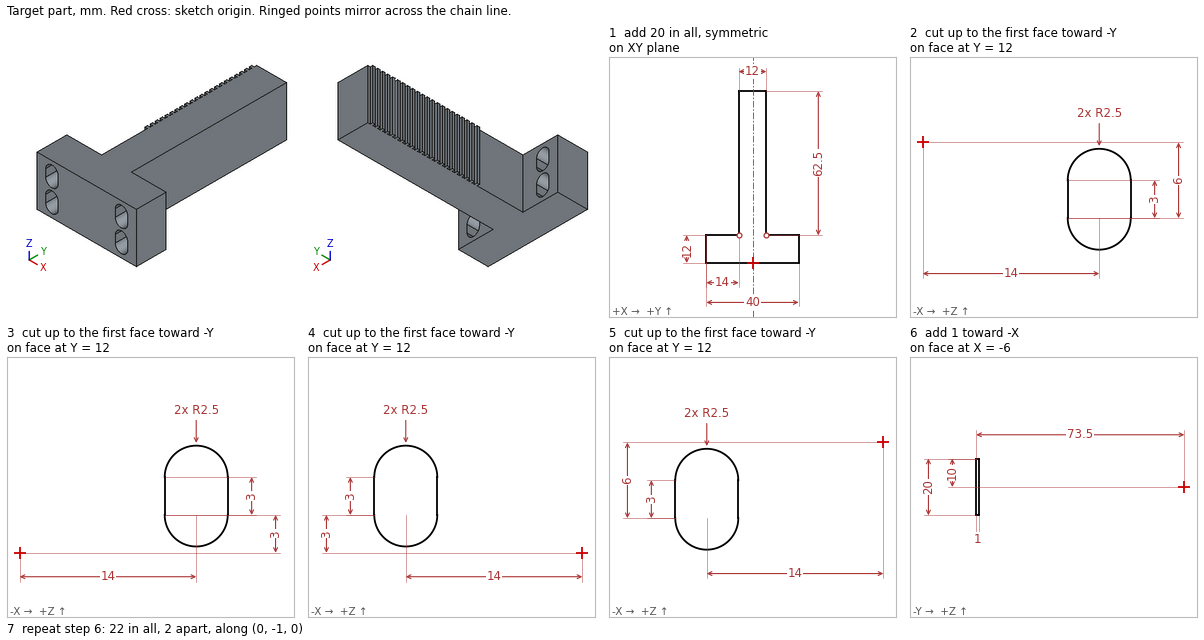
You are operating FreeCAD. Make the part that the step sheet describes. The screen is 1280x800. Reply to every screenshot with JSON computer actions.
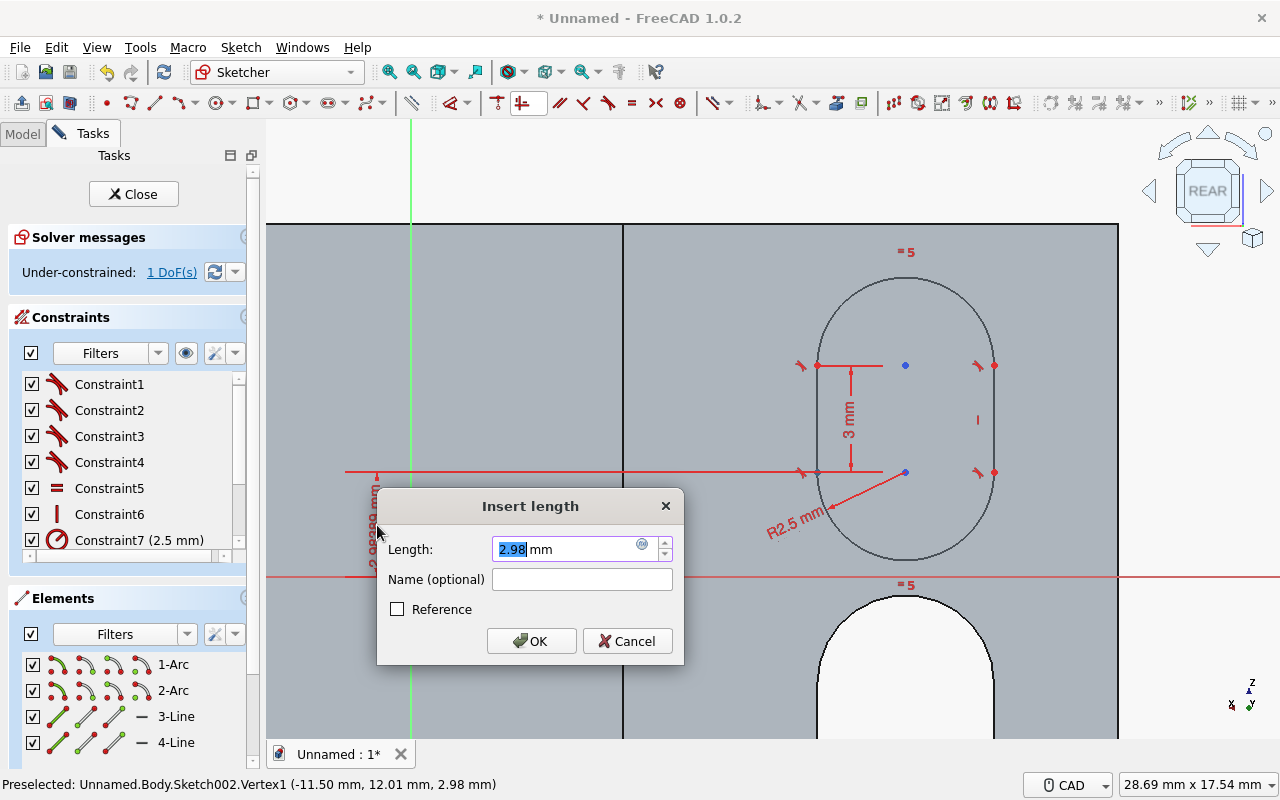
{"action": "type", "text": "3"}
{"action": "key", "text": "Return"}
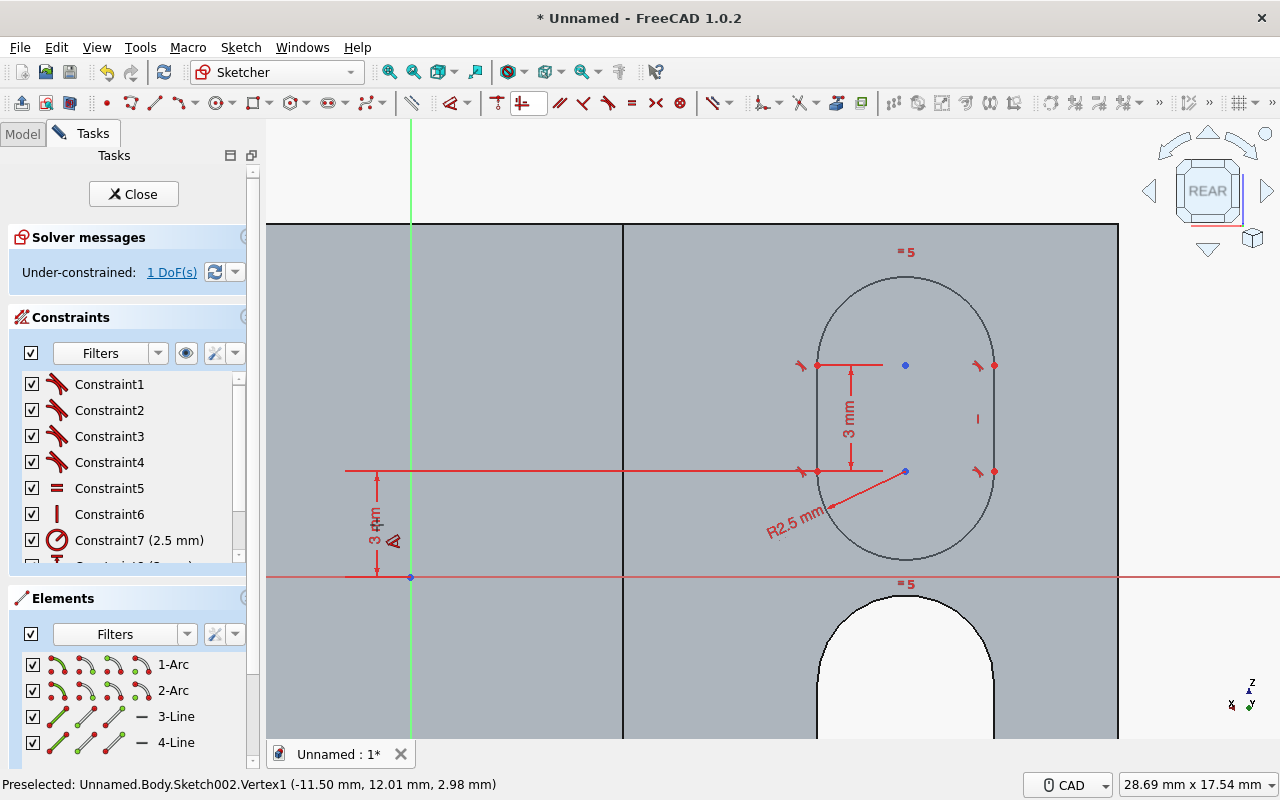
{"action": "left_click", "coordinate": [906, 471]}
{"action": "left_click", "coordinate": [658, 611]}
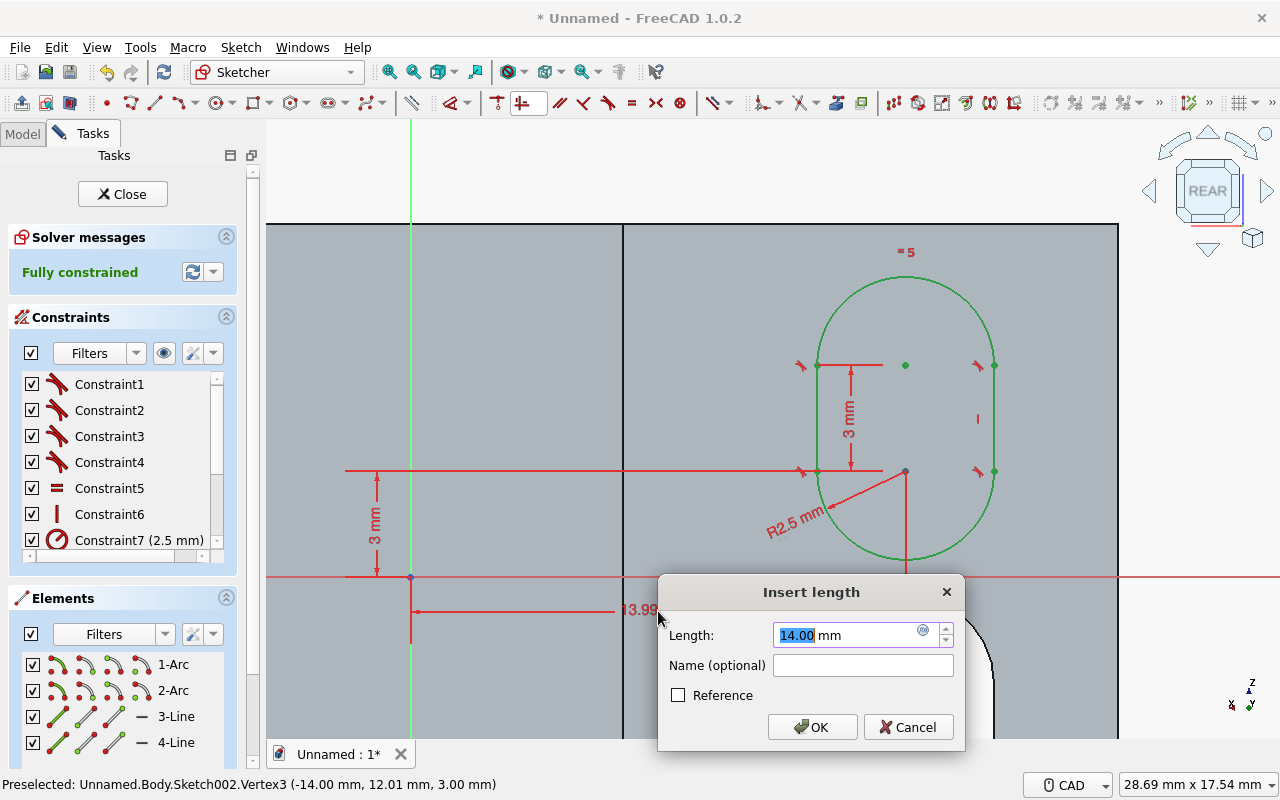
{"action": "type", "text": "14"}
{"action": "key", "text": "Return"}
{"action": "key", "text": "Escape"}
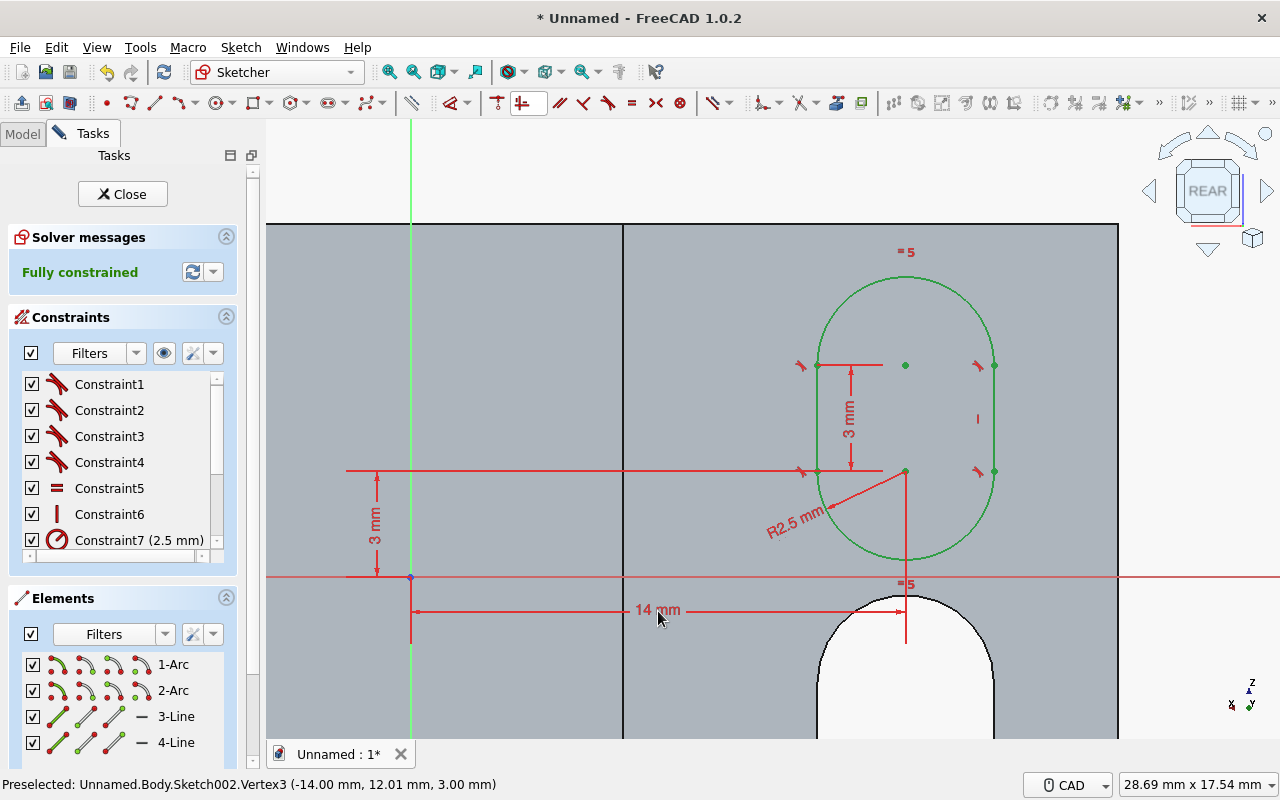
{"action": "left_click", "coordinate": [123, 194]}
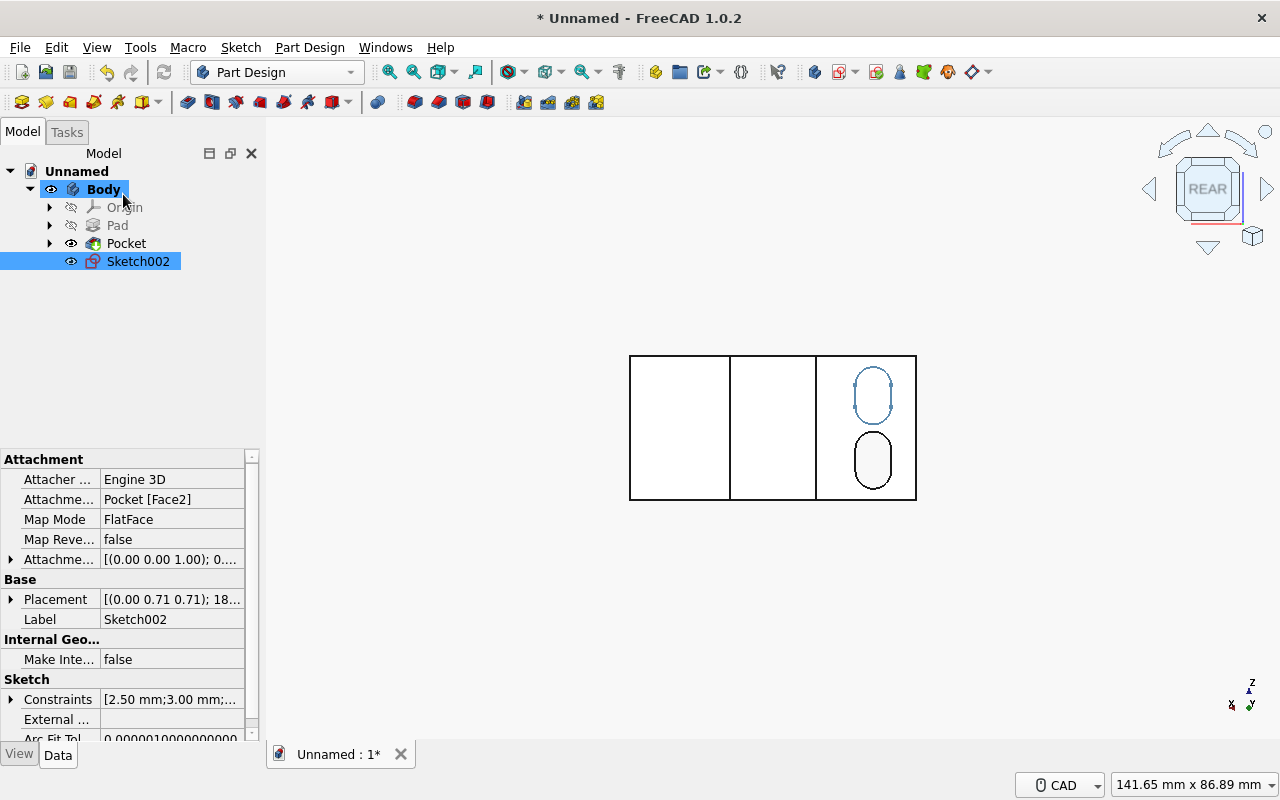
{"action": "left_click", "coordinate": [188, 102]}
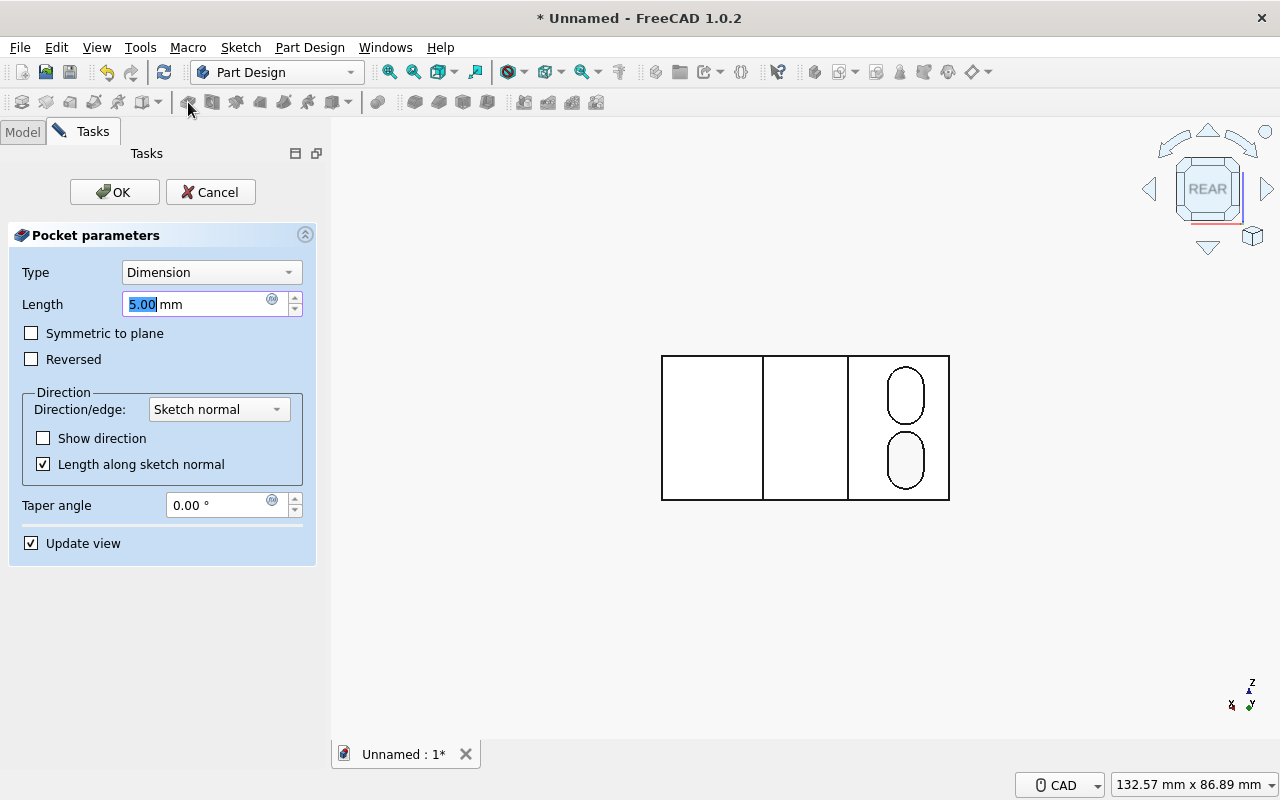
{"action": "left_click", "coordinate": [212, 272]}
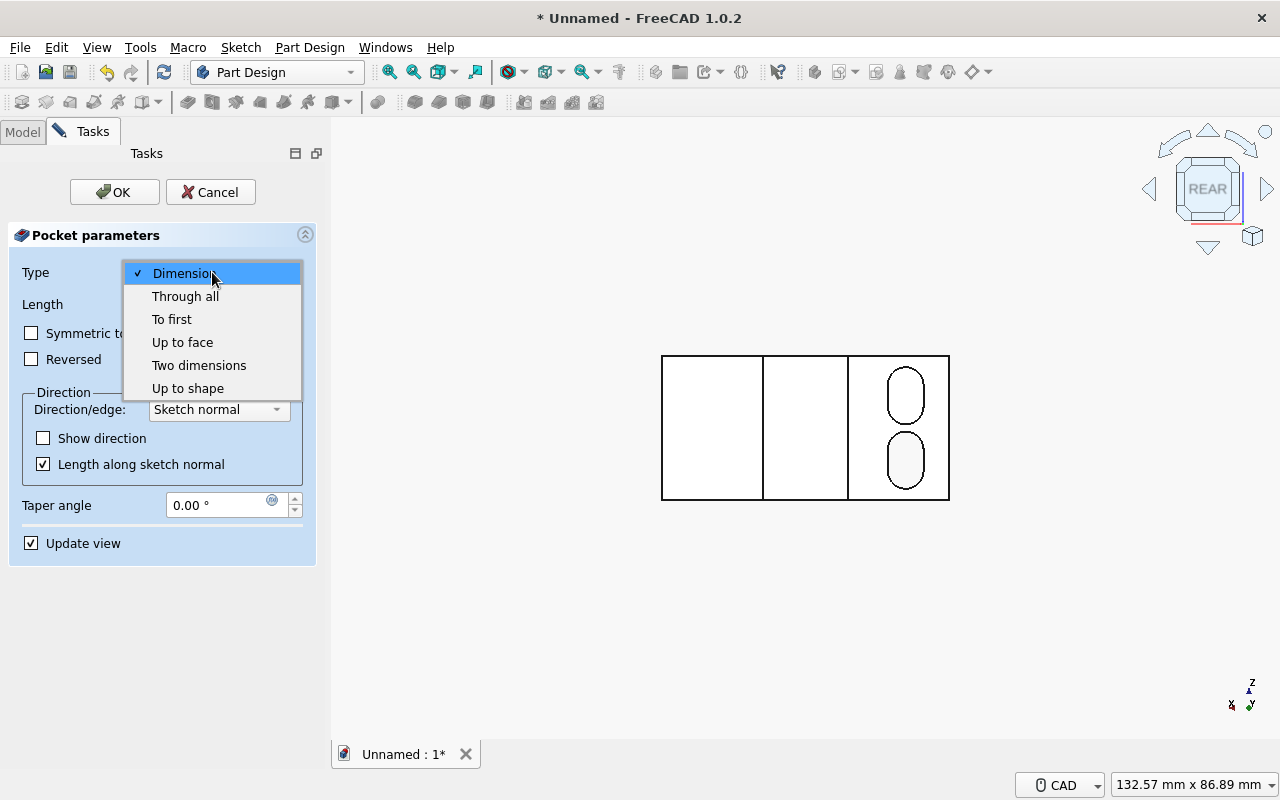
{"action": "left_click", "coordinate": [212, 320]}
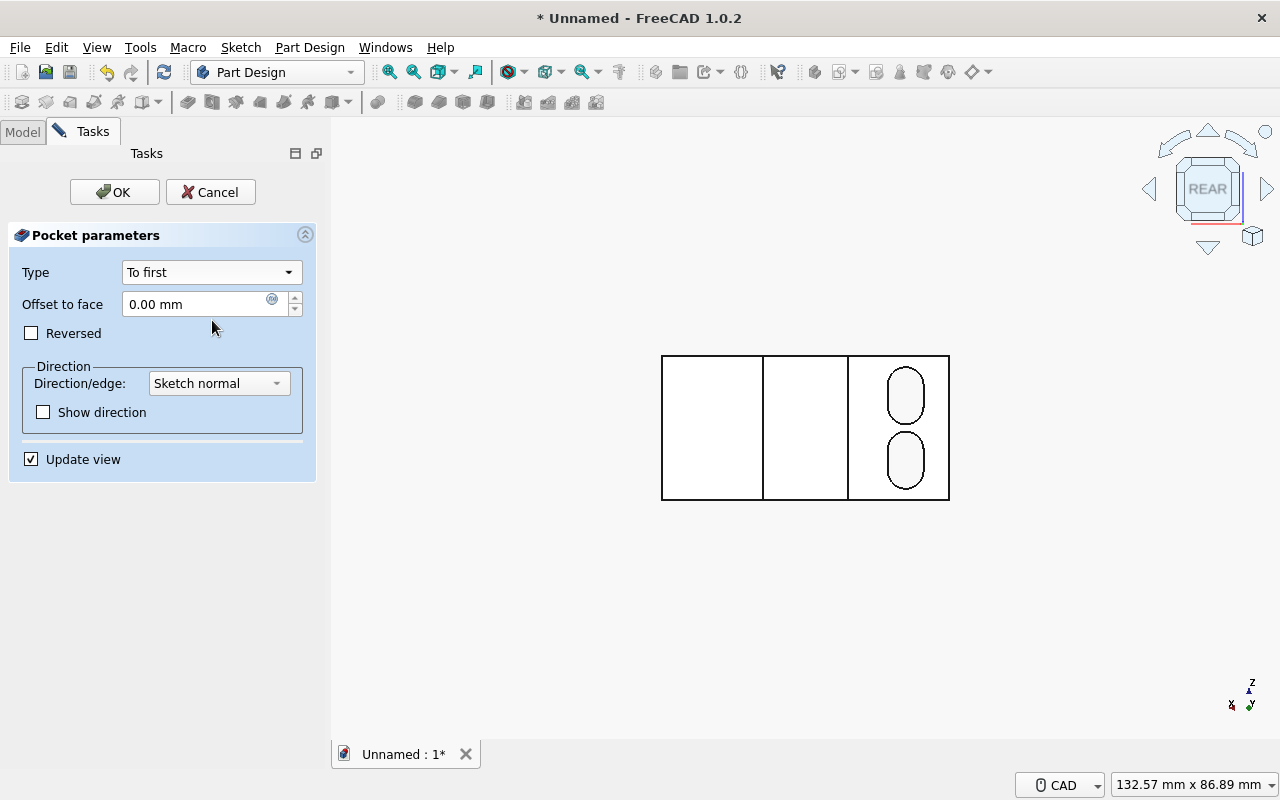
{"action": "left_click", "coordinate": [115, 192]}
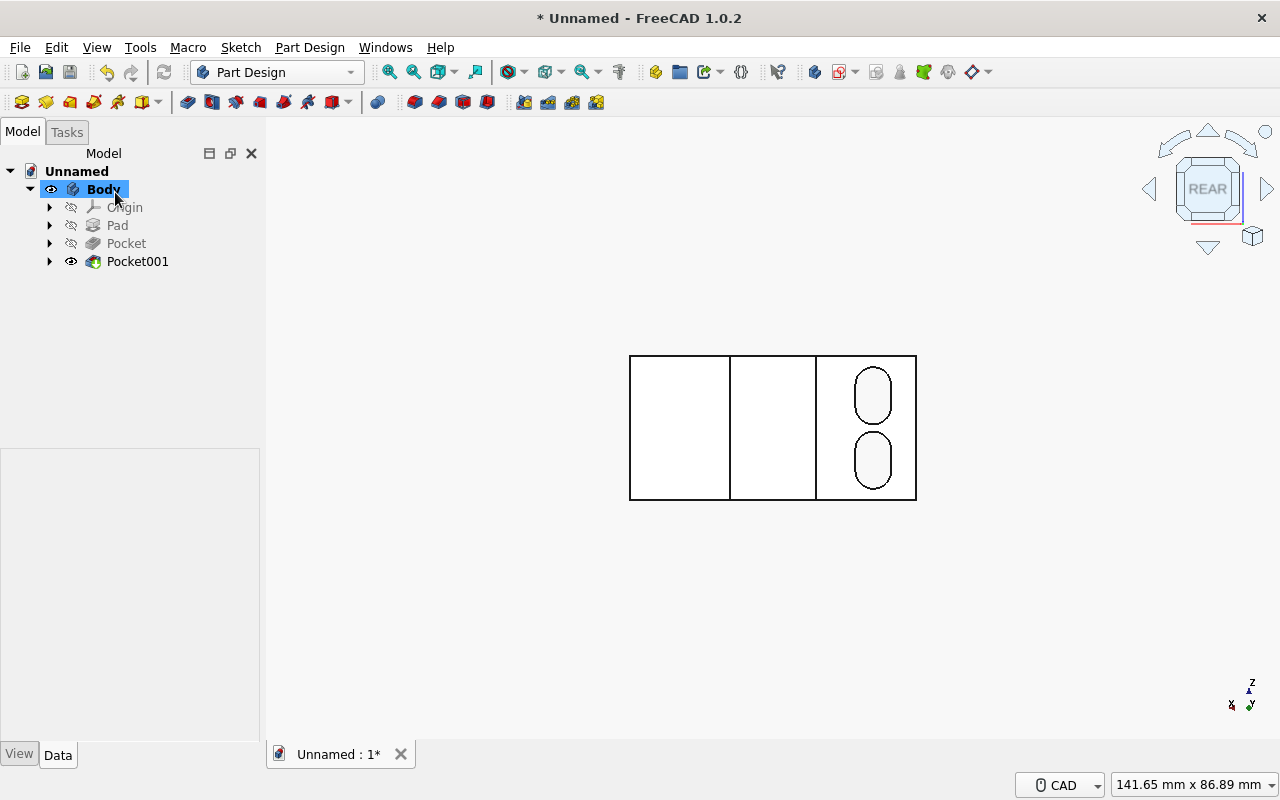
{"action": "left_click", "coordinate": [390, 72]}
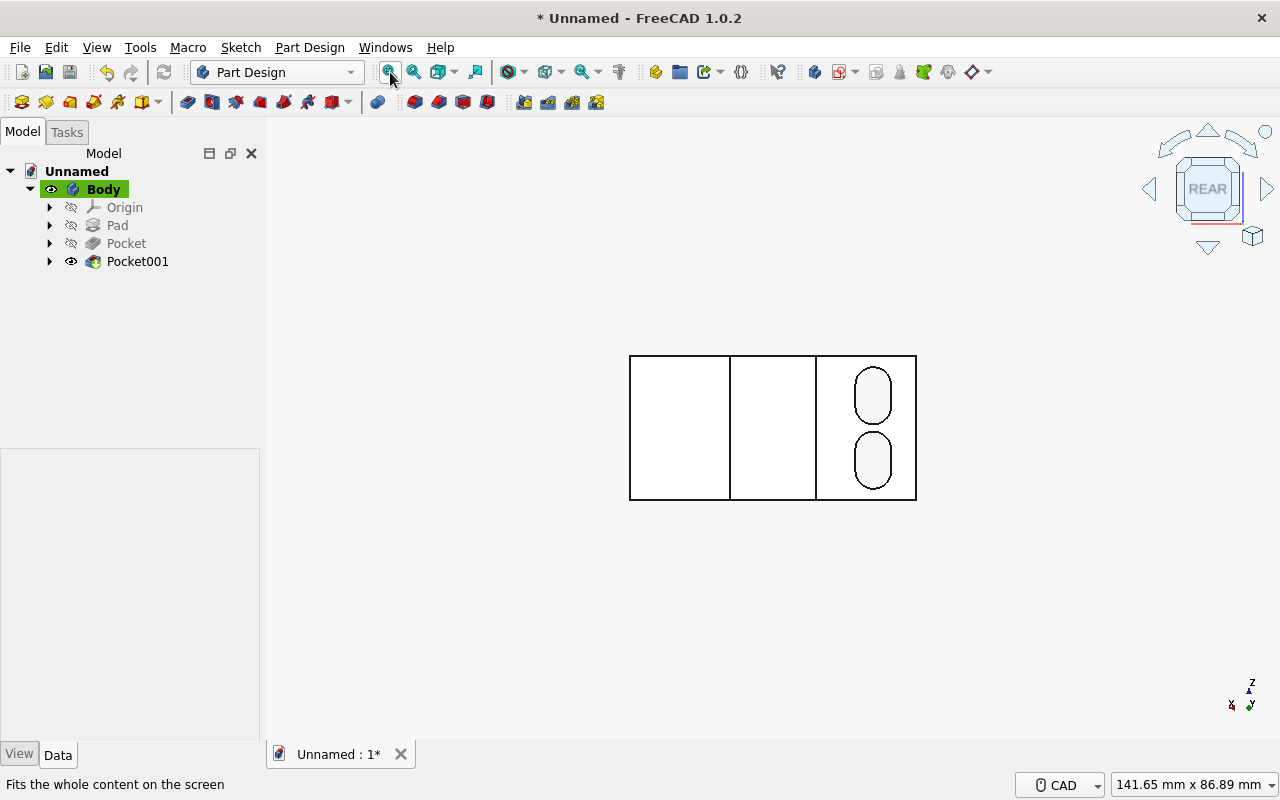
{"action": "left_click", "coordinate": [680, 407]}